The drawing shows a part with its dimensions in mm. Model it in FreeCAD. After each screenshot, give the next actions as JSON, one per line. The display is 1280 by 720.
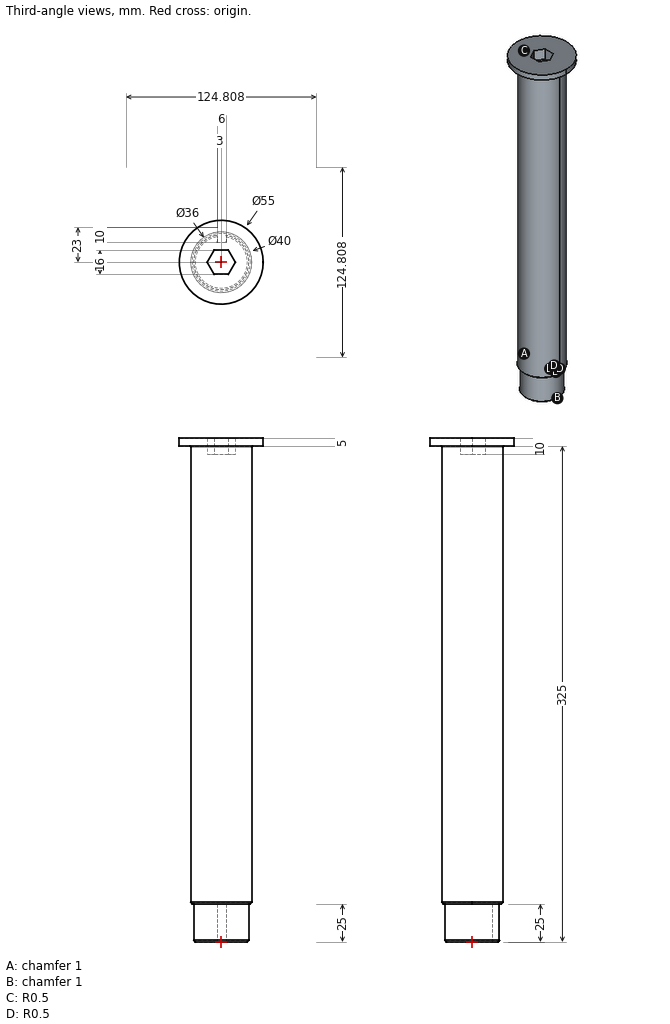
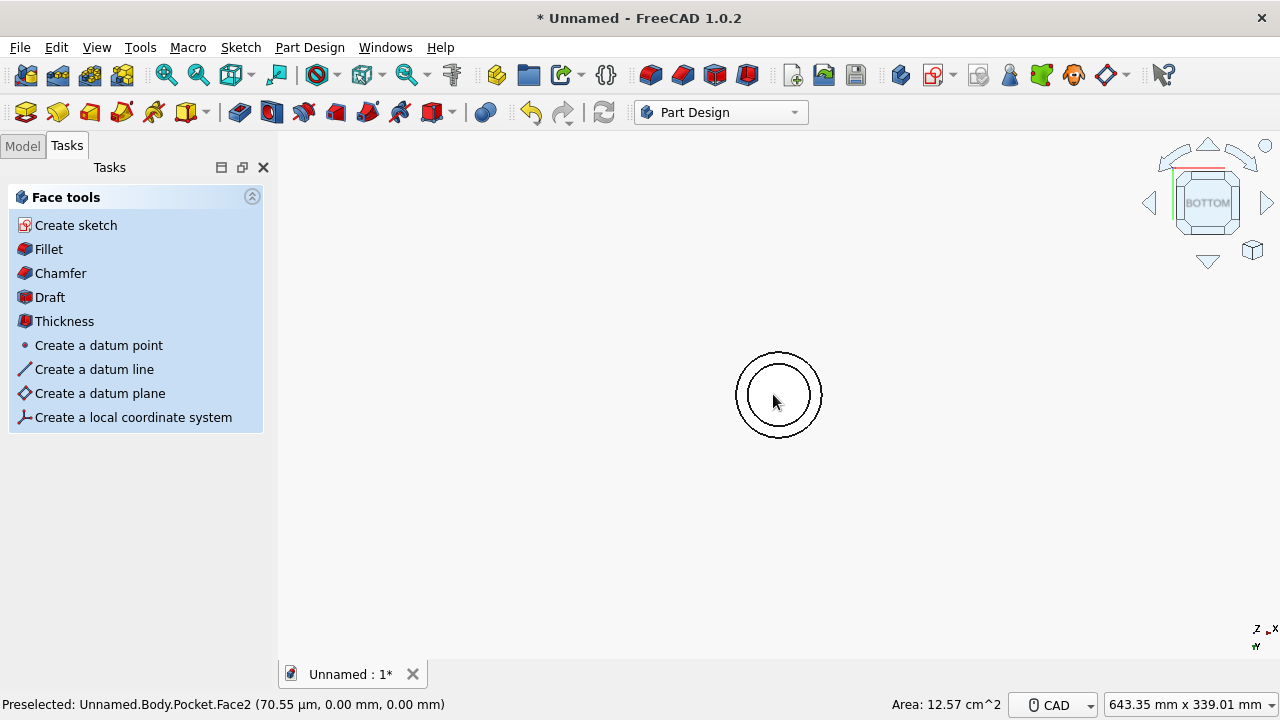
{"action": "left_click", "coordinate": [934, 76]}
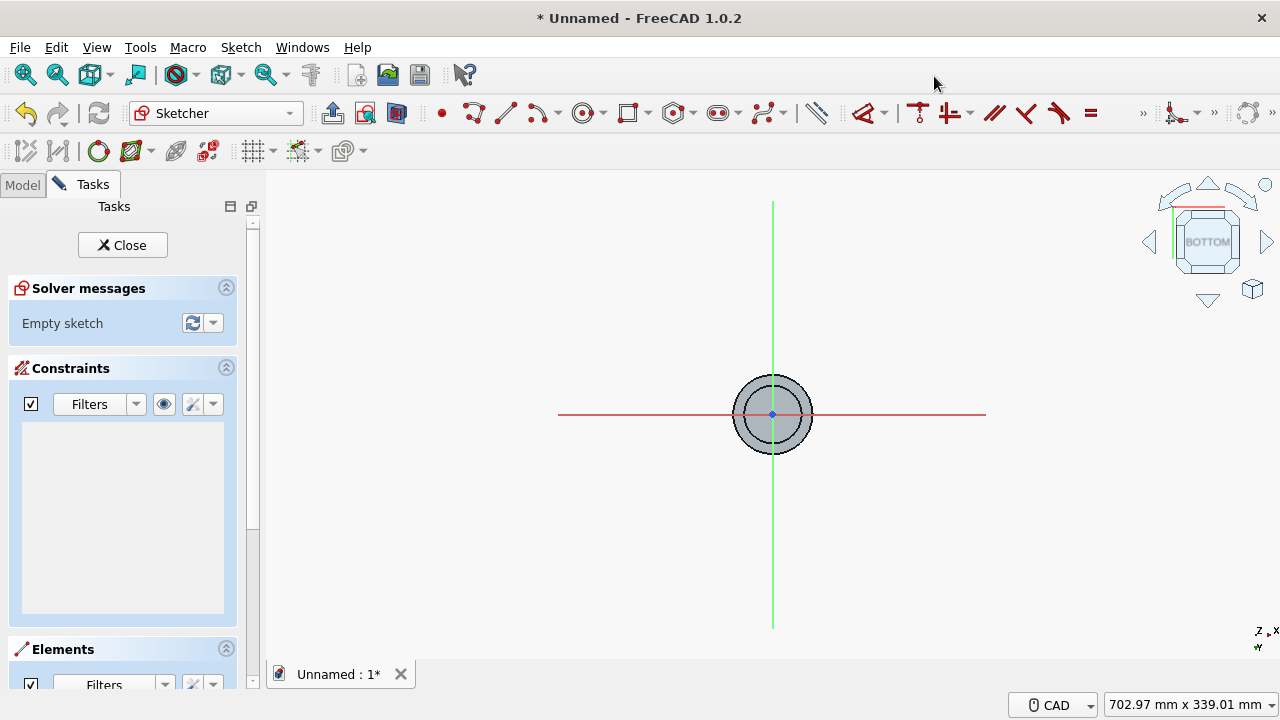
{"action": "scroll", "coordinate": [856, 415], "scroll_direction": "up", "scroll_amount": 3}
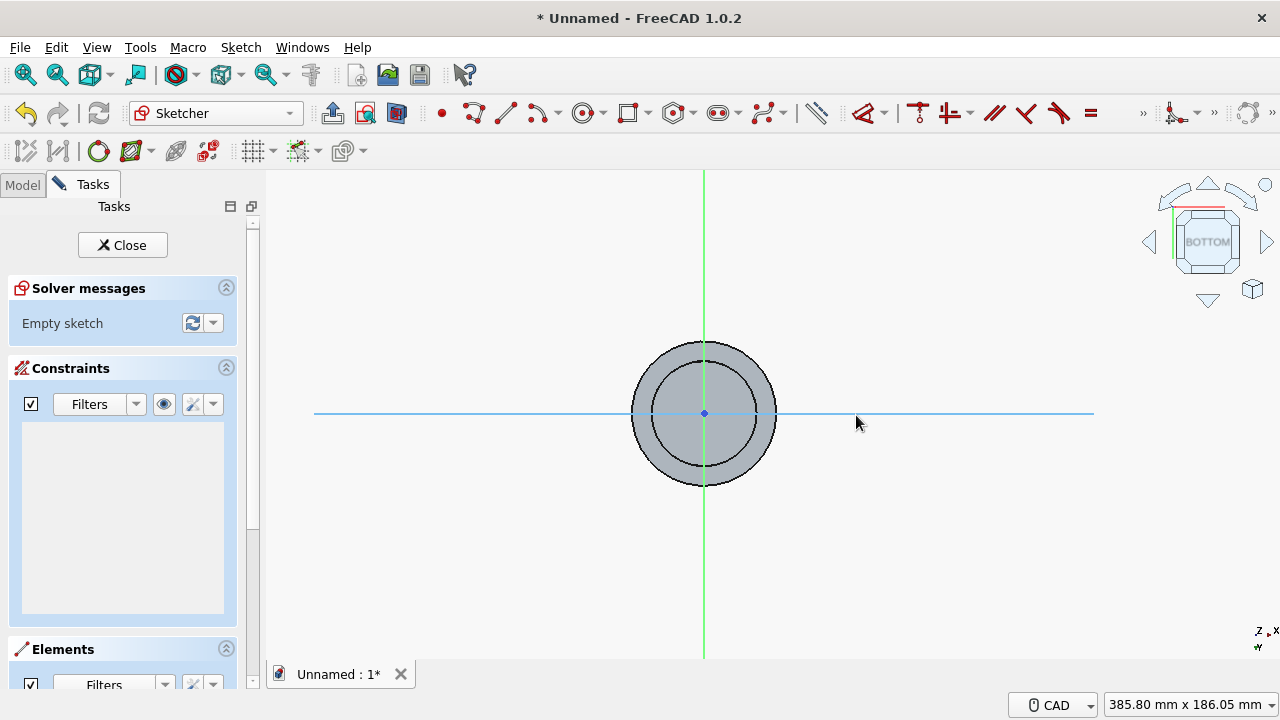
{"action": "key", "text": "g v"}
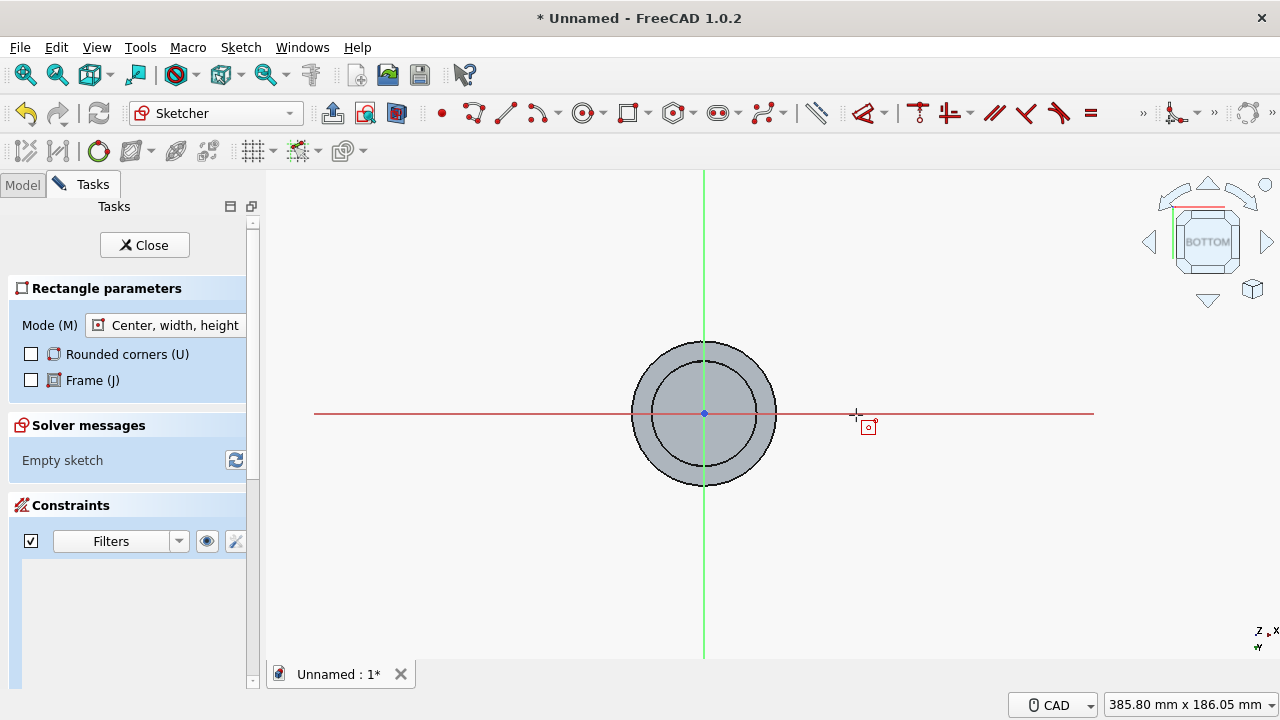
{"action": "left_click", "coordinate": [704, 414]}
{"action": "left_click", "coordinate": [868, 250]}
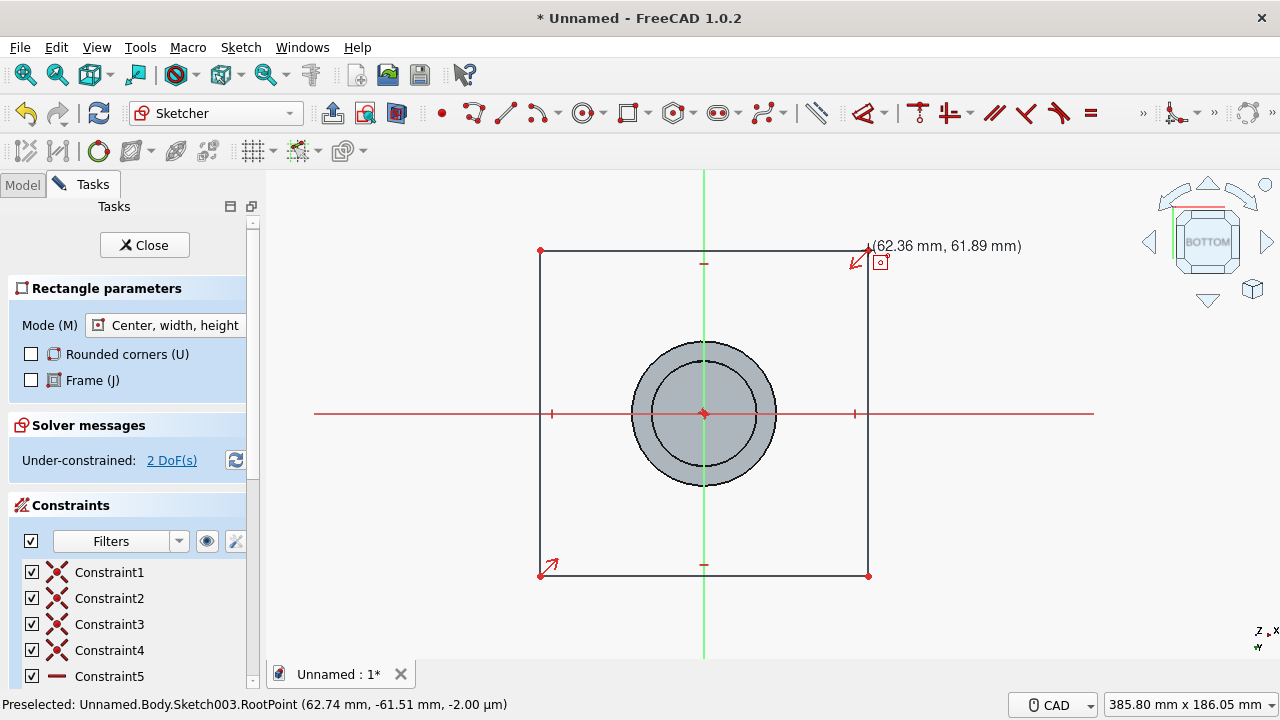
{"action": "left_click", "coordinate": [584, 114]}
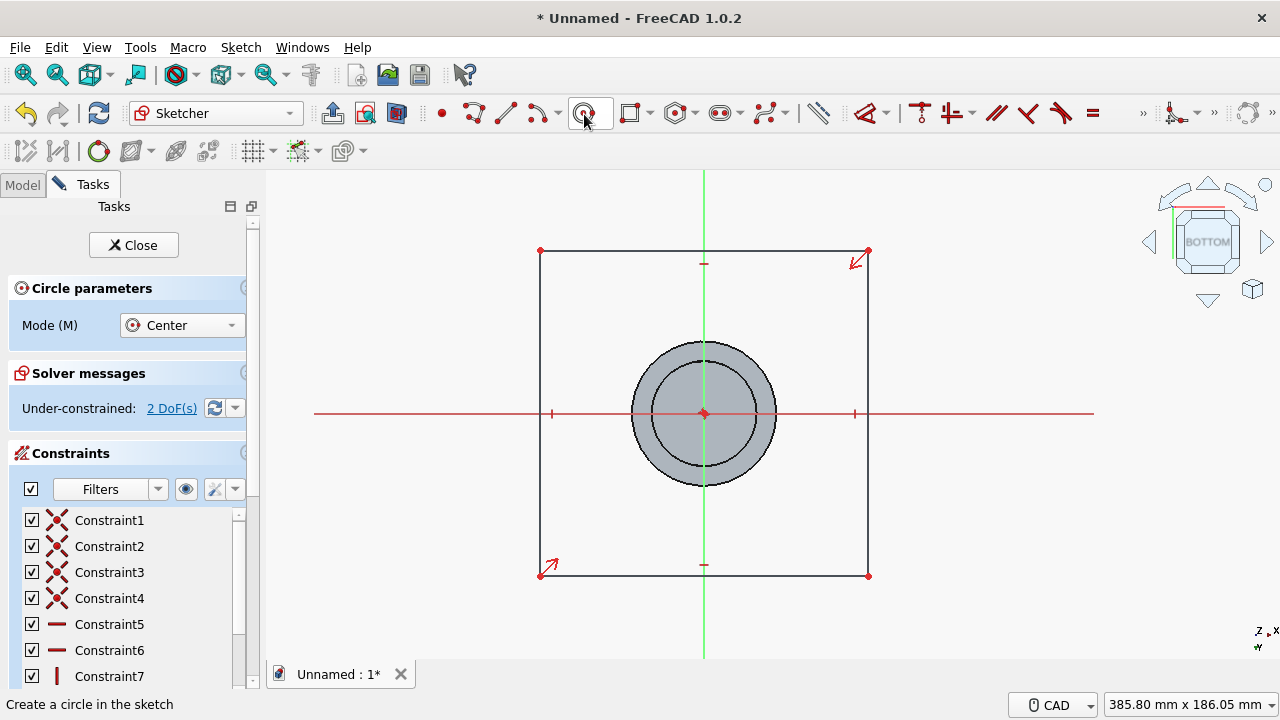
{"action": "left_click", "coordinate": [704, 414]}
{"action": "left_click", "coordinate": [738, 380]}
{"action": "key", "text": "Escape"}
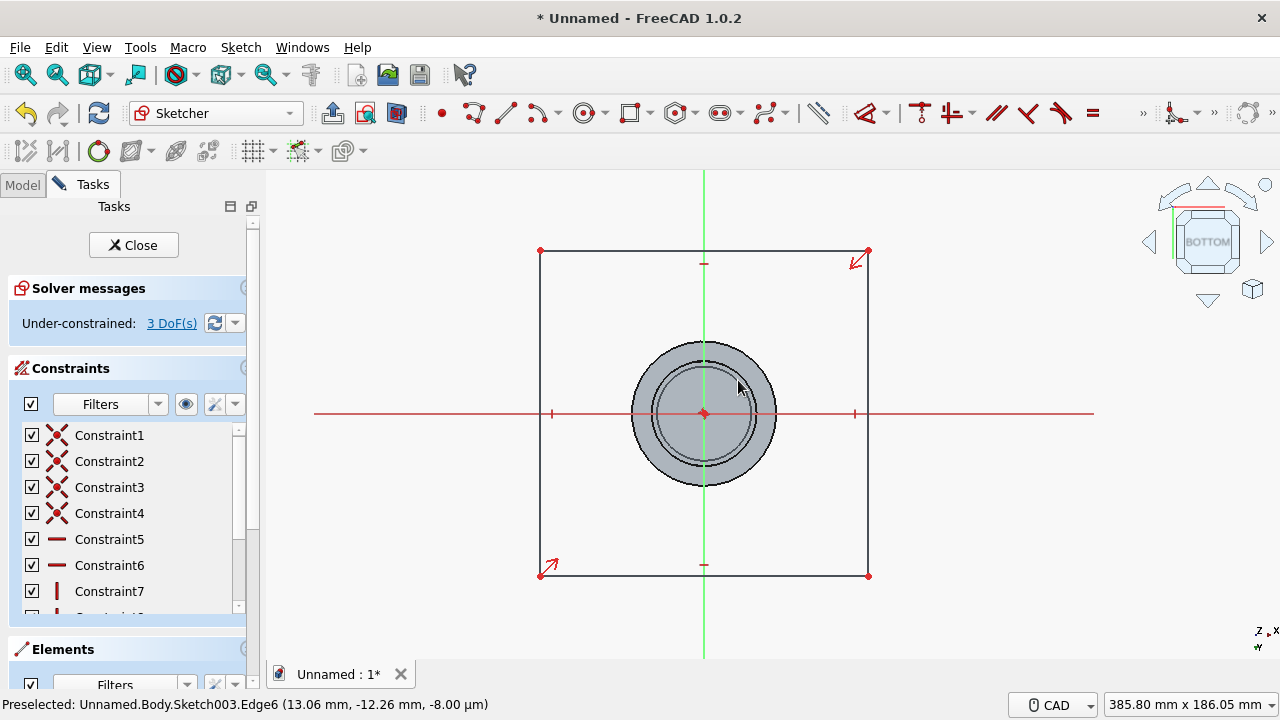
{"action": "left_click", "coordinate": [866, 114]}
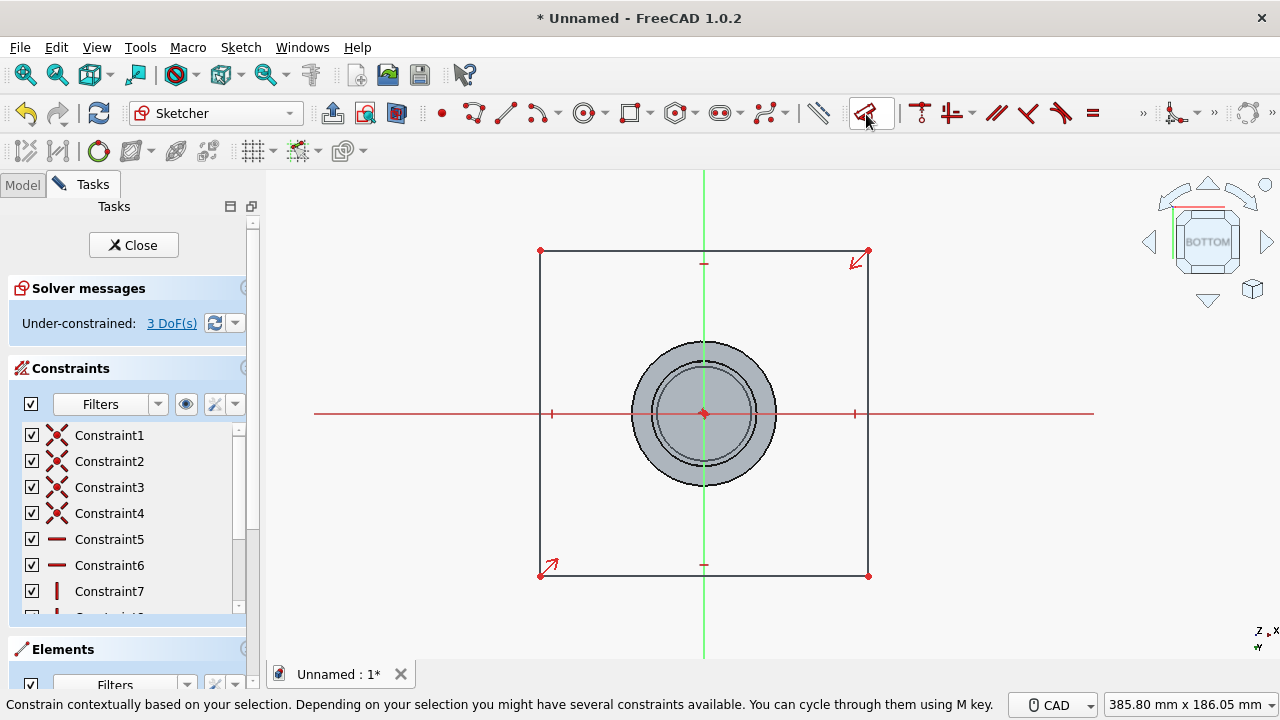
{"action": "left_click", "coordinate": [737, 380]}
{"action": "left_click", "coordinate": [759, 357]}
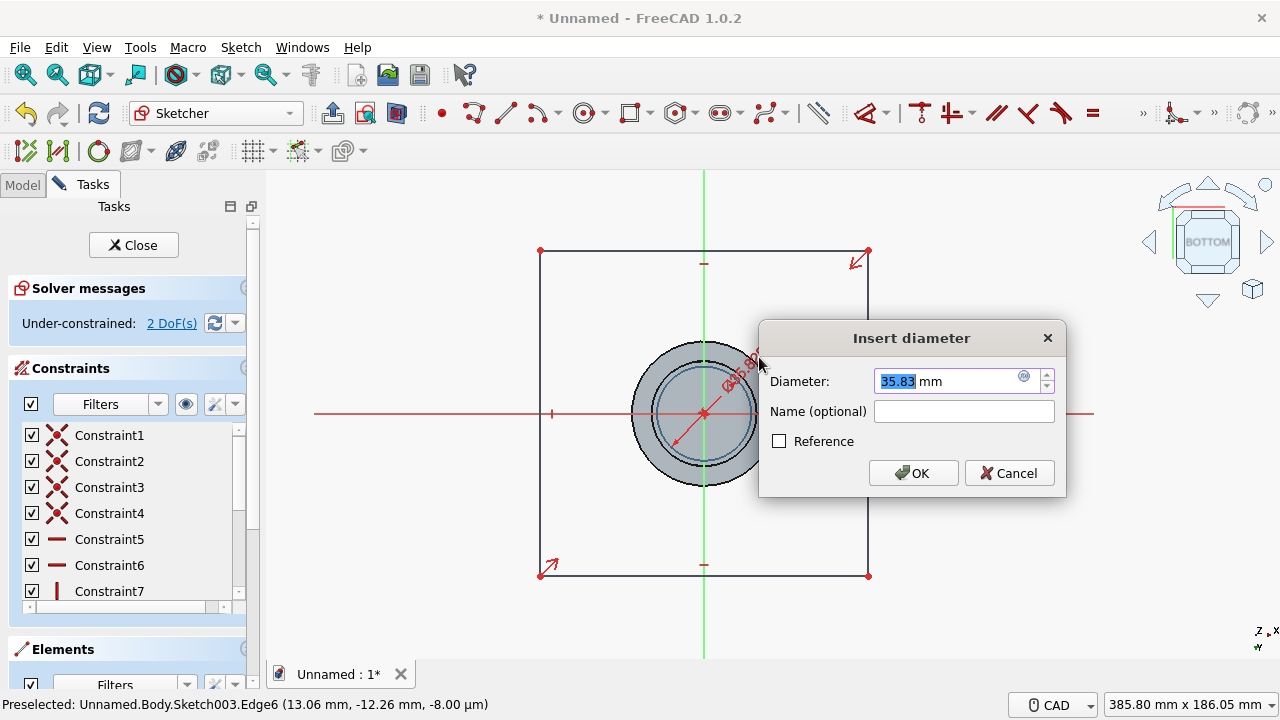
{"action": "type", "text": "36"}
{"action": "key", "text": "Return"}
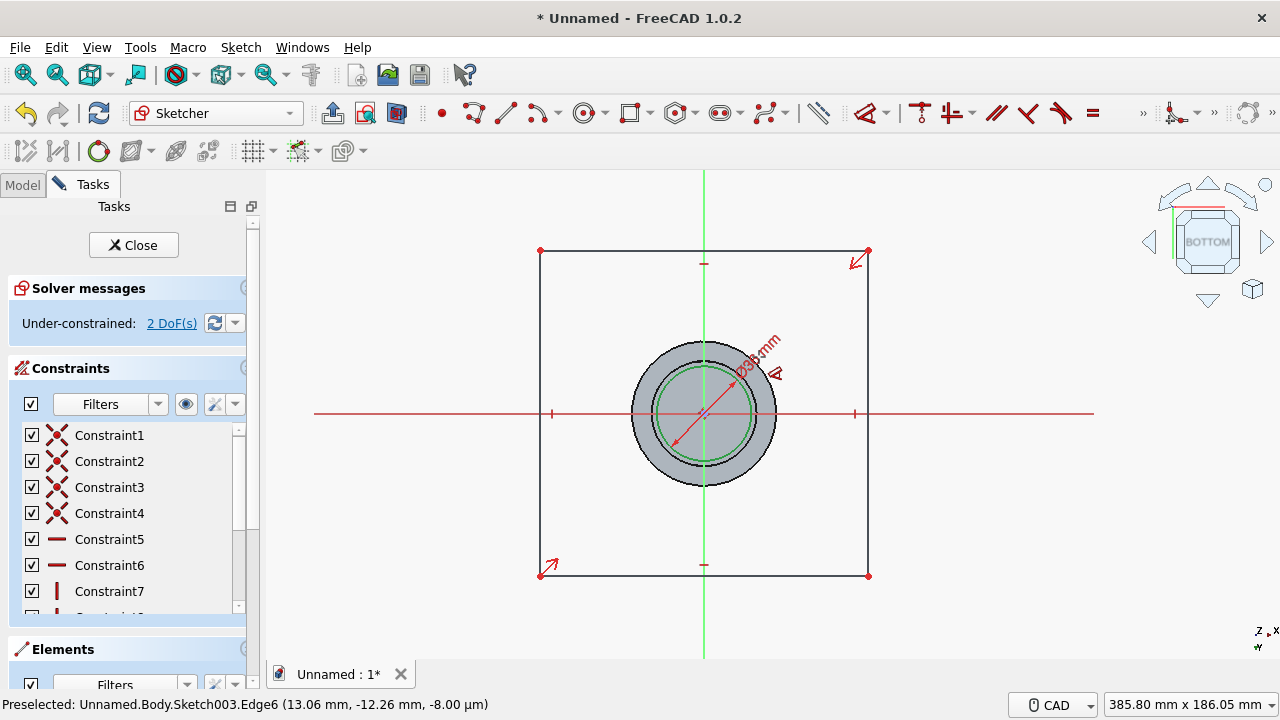
{"action": "left_click", "coordinate": [639, 576]}
{"action": "left_click", "coordinate": [629, 610]}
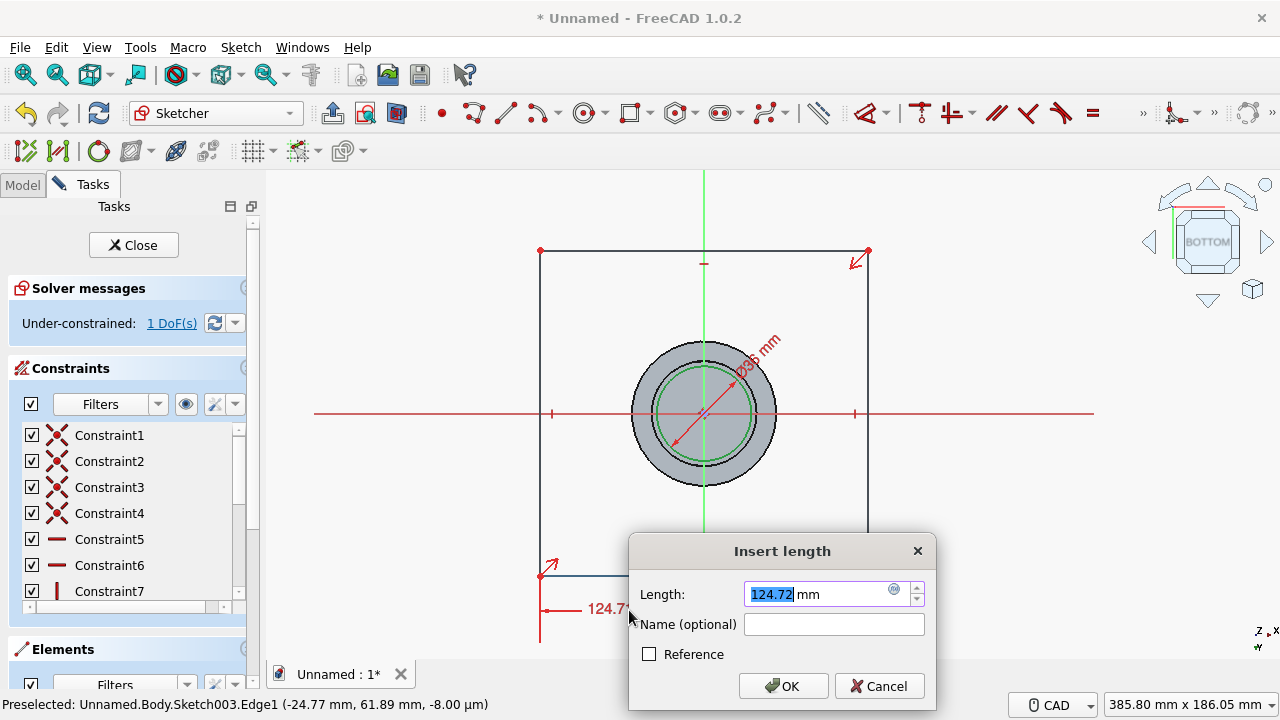
{"action": "type", "text": "124.808"}
{"action": "key", "text": "Return"}